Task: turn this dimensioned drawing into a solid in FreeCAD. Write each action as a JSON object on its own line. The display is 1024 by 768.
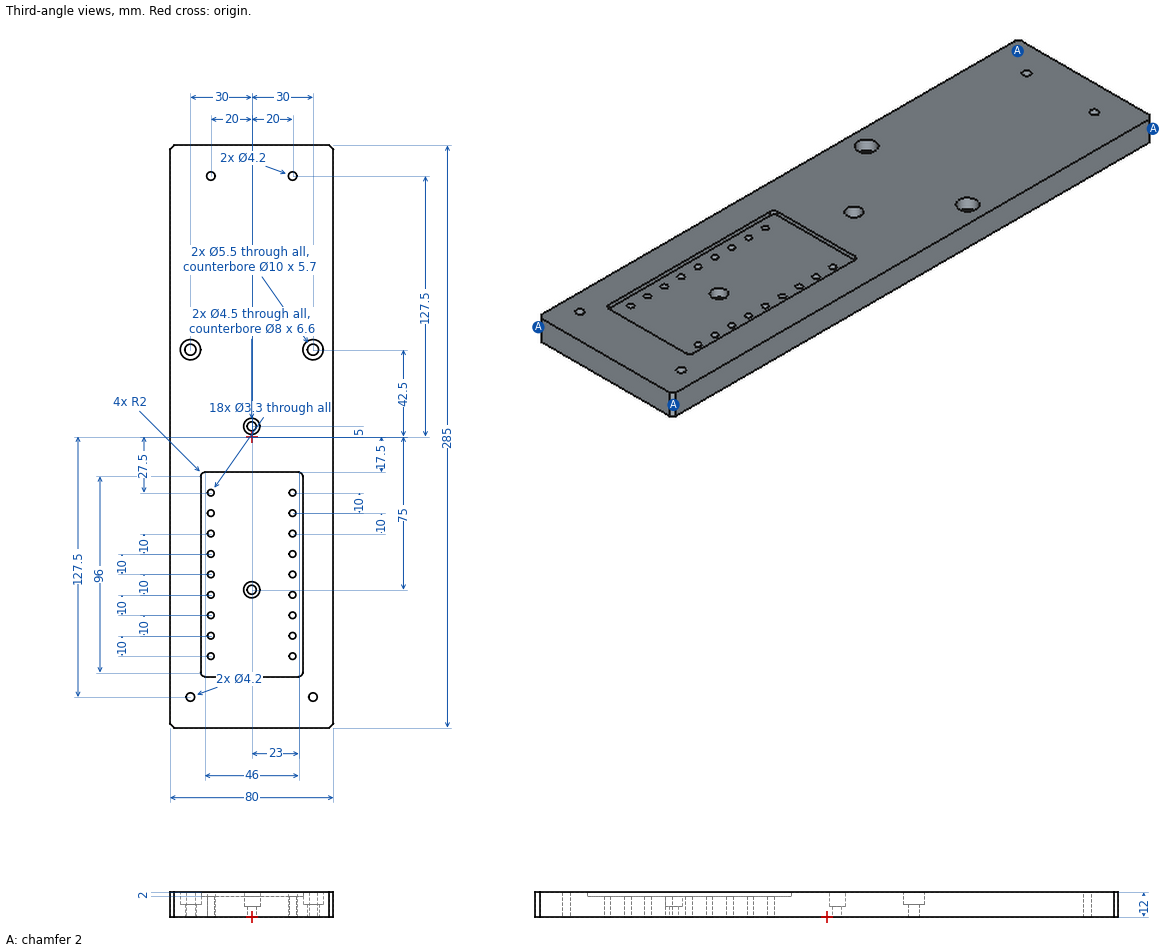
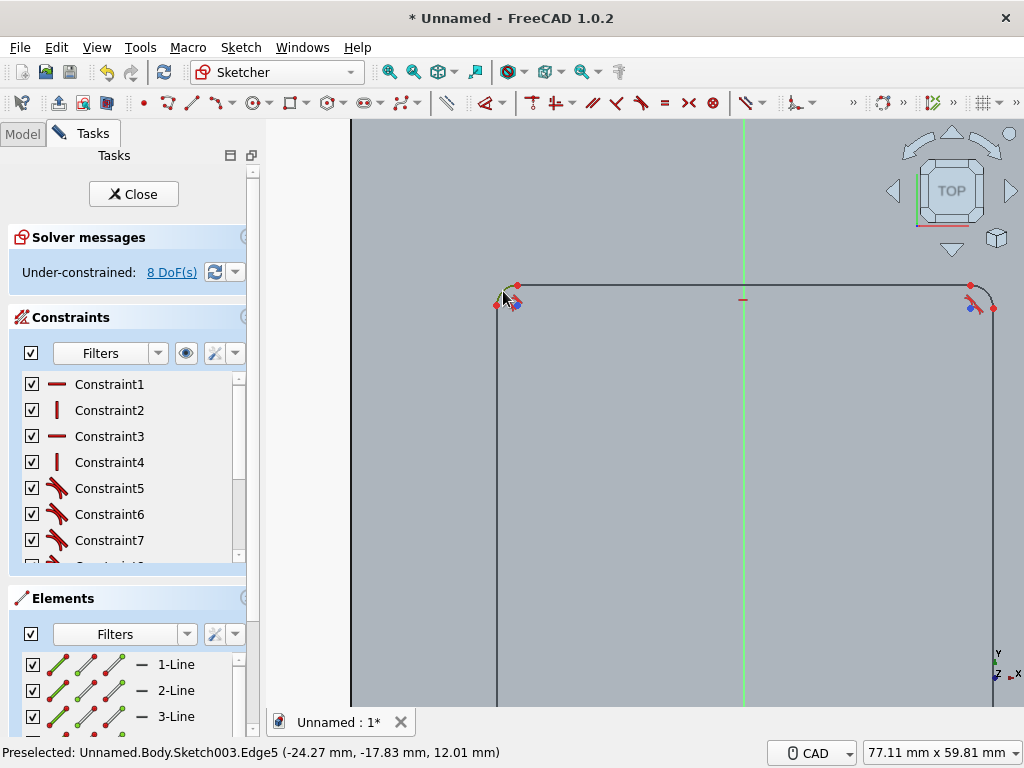
{"action": "scroll", "coordinate": [504, 293], "scroll_direction": "down", "scroll_amount": 6}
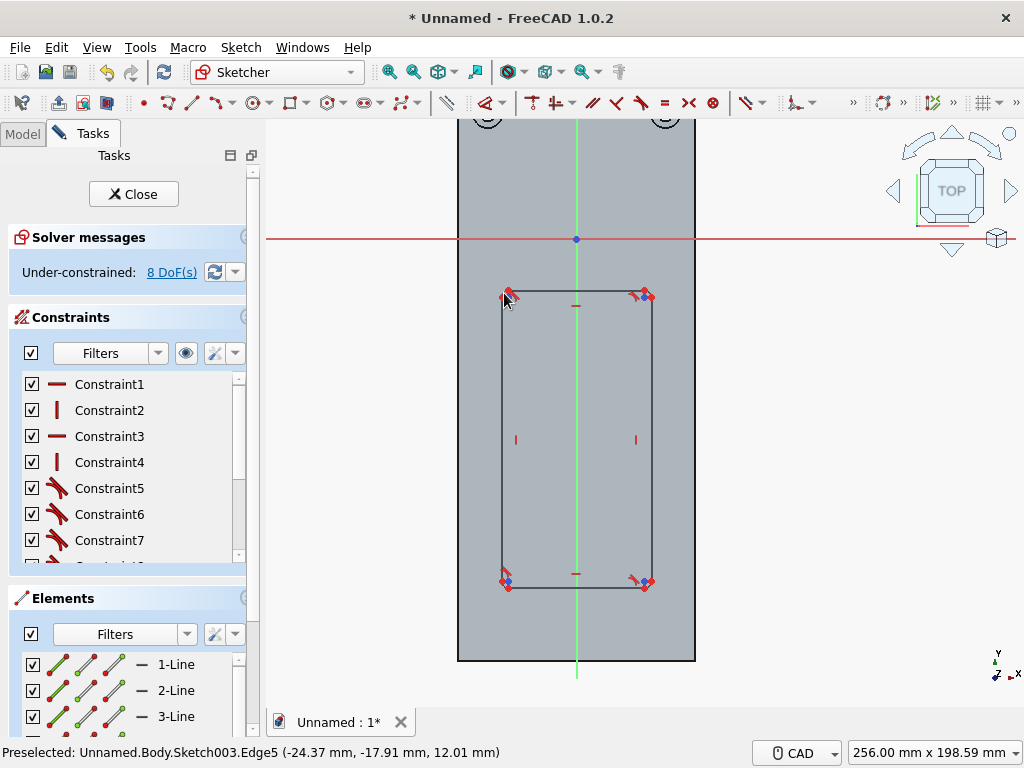
{"action": "scroll", "coordinate": [503, 585], "scroll_direction": "up", "scroll_amount": 8}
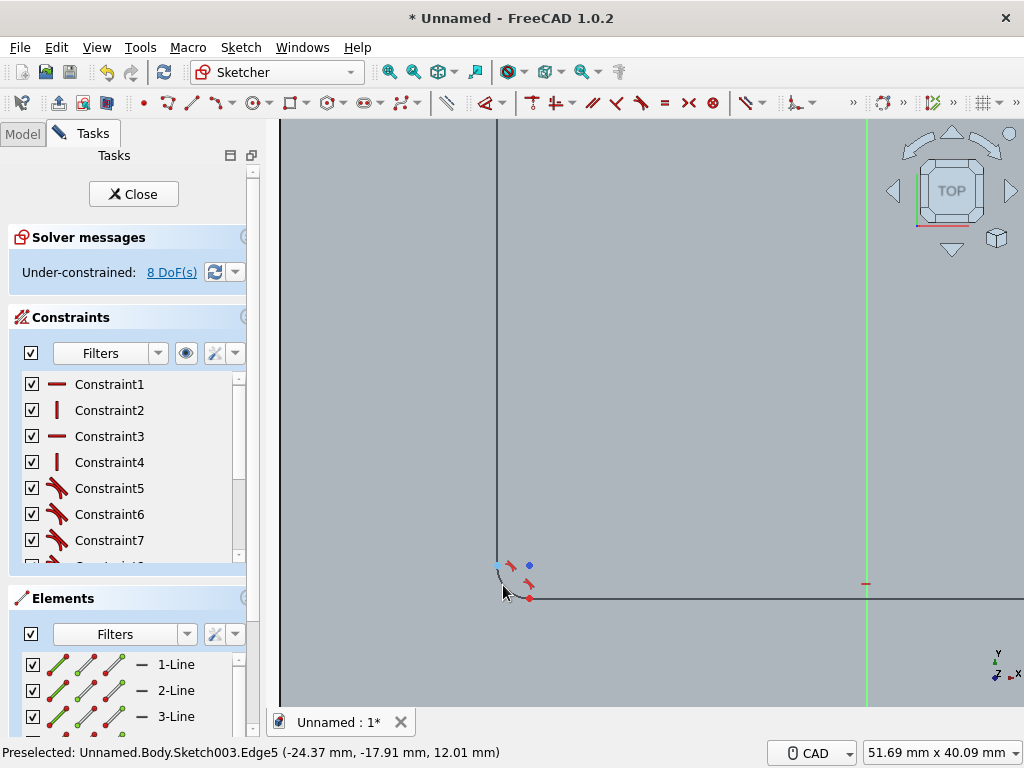
{"action": "left_click", "coordinate": [501, 581]}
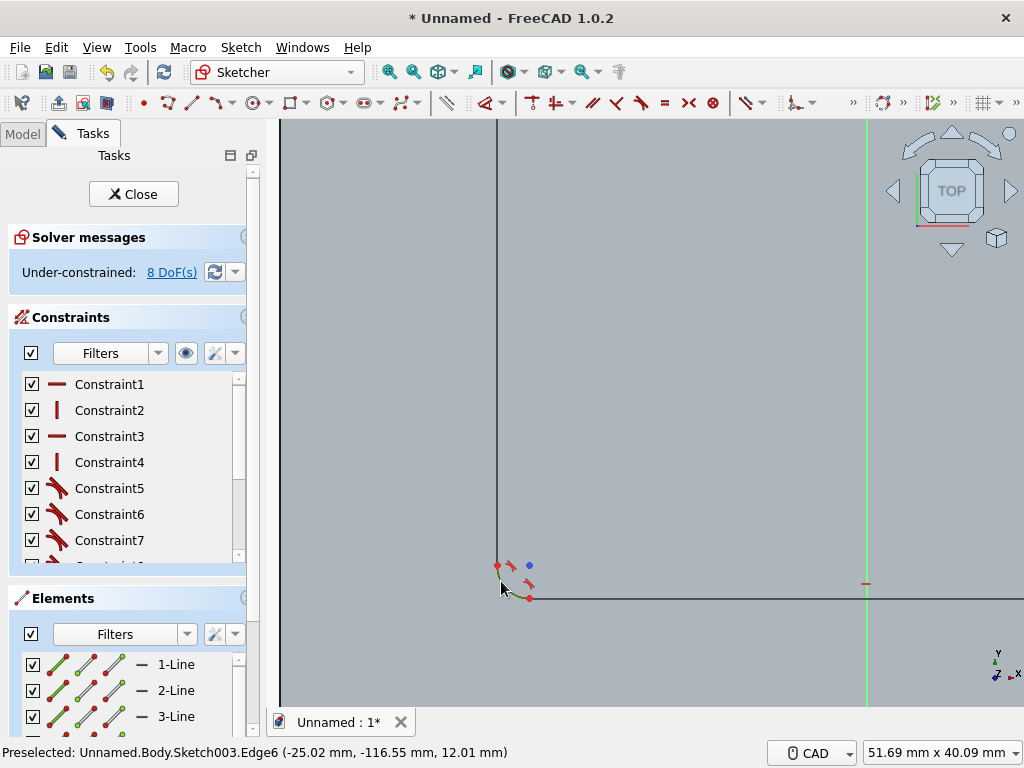
{"action": "scroll", "coordinate": [503, 586], "scroll_direction": "down", "scroll_amount": 8}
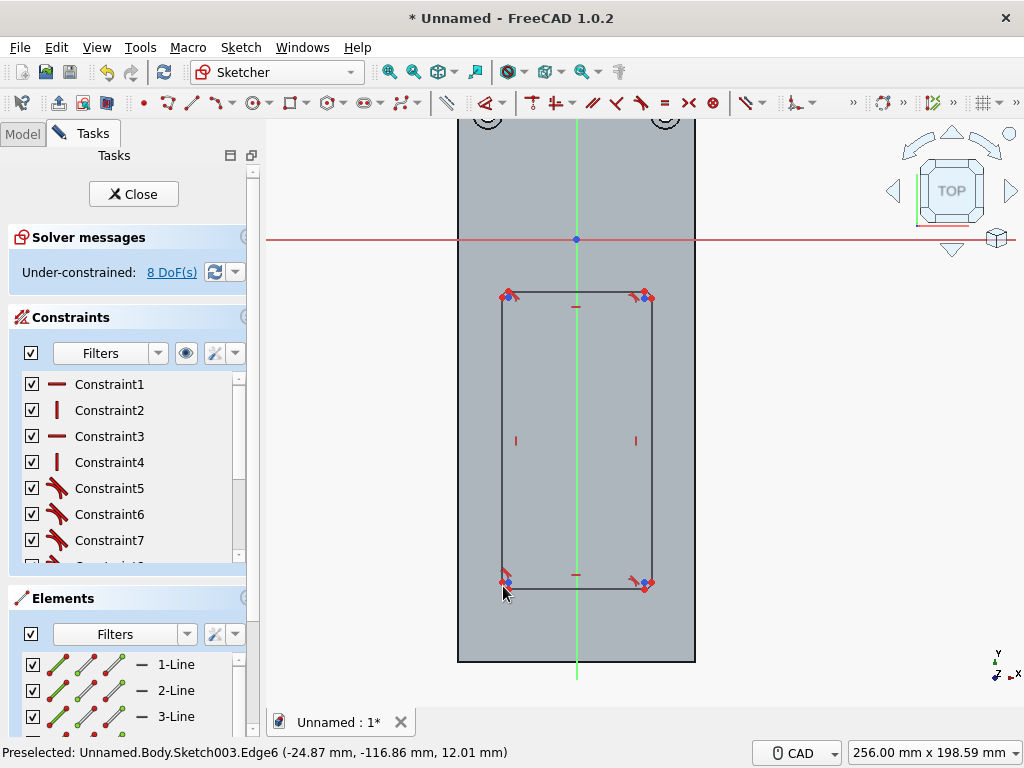
{"action": "scroll", "coordinate": [648, 588], "scroll_direction": "up", "scroll_amount": 8}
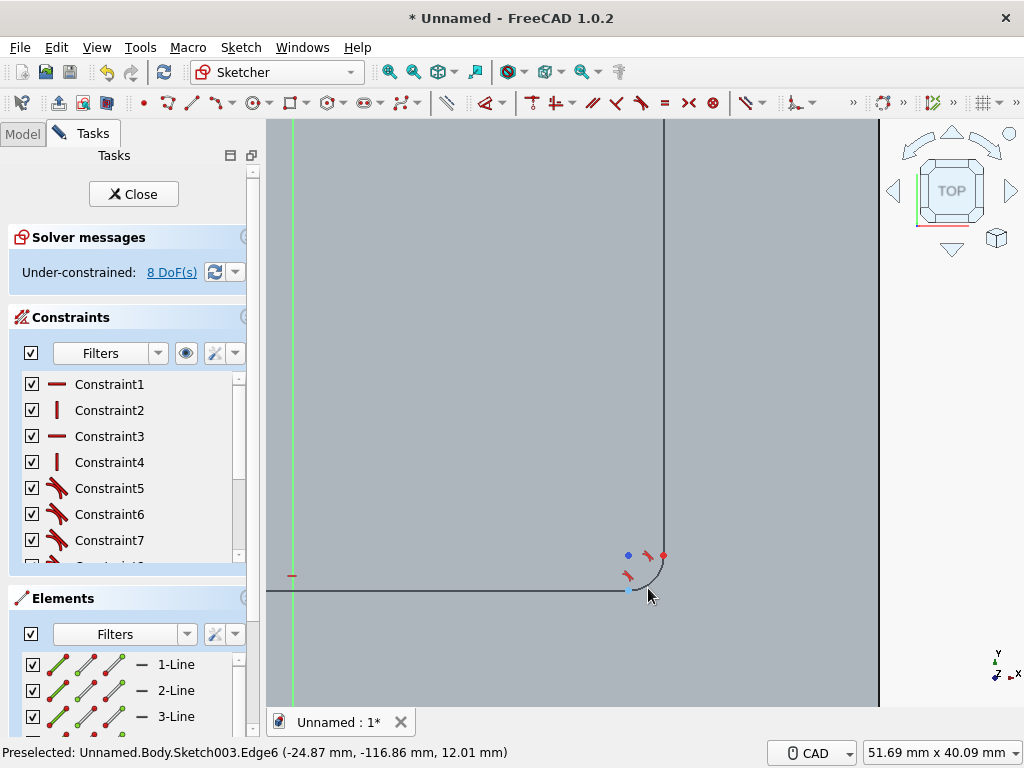
{"action": "left_click", "coordinate": [645, 587]}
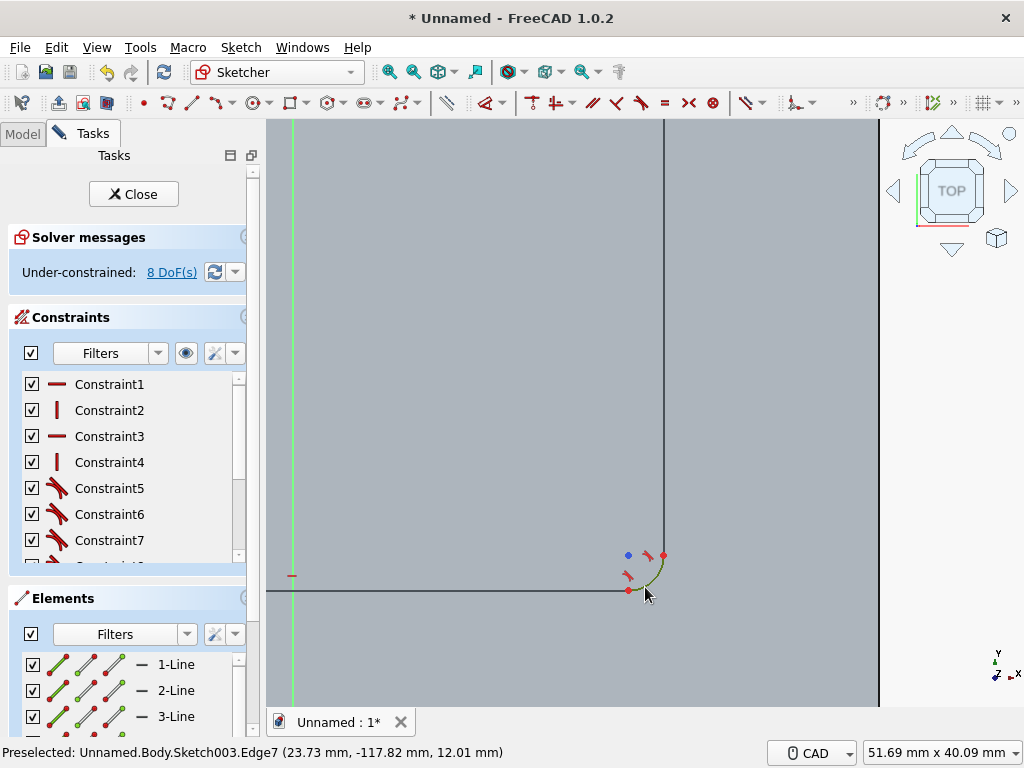
{"action": "scroll", "coordinate": [648, 588], "scroll_direction": "down", "scroll_amount": 8}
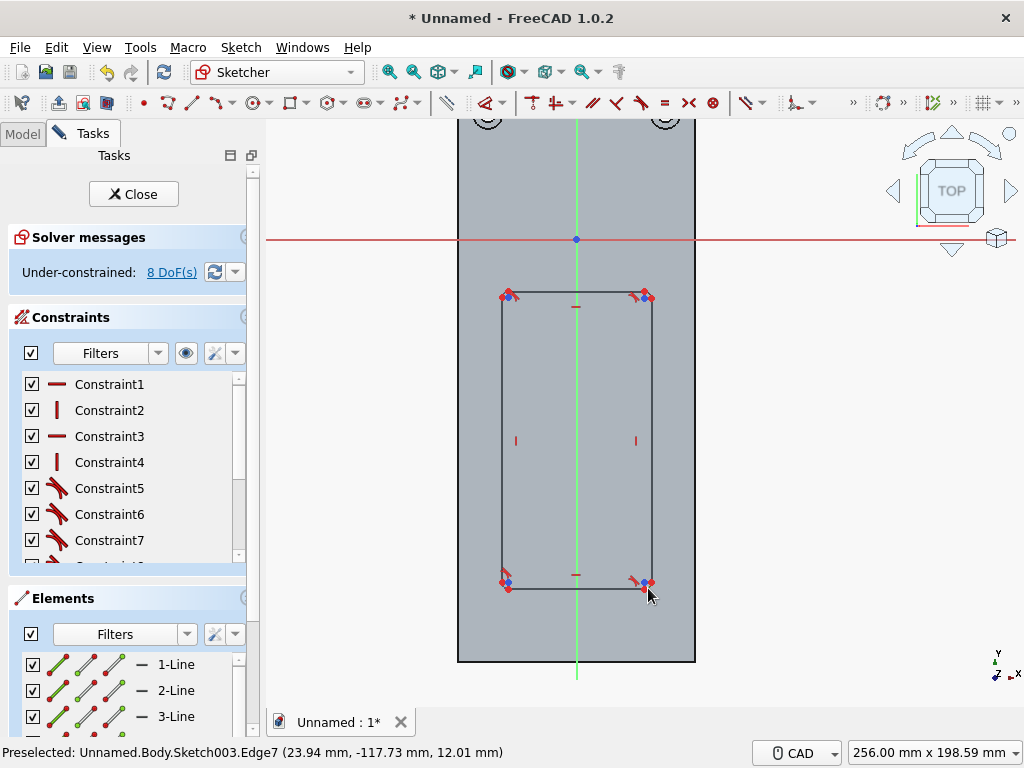
{"action": "scroll", "coordinate": [651, 295], "scroll_direction": "up", "scroll_amount": 8}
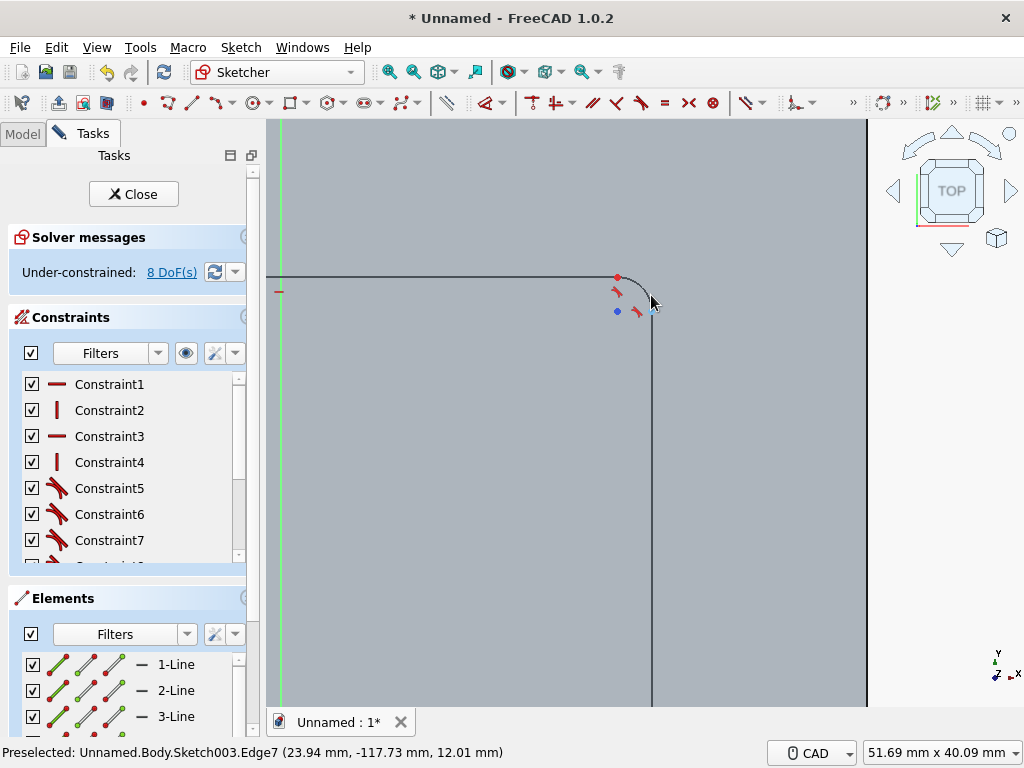
{"action": "left_click", "coordinate": [648, 296]}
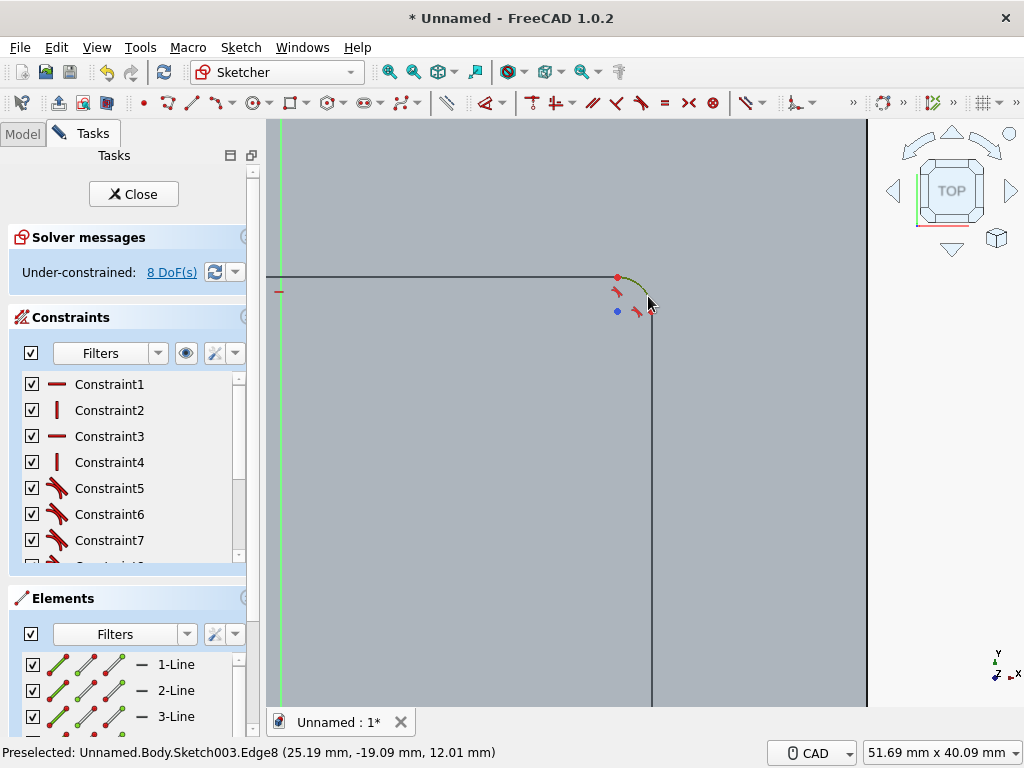
{"action": "key", "text": "e"}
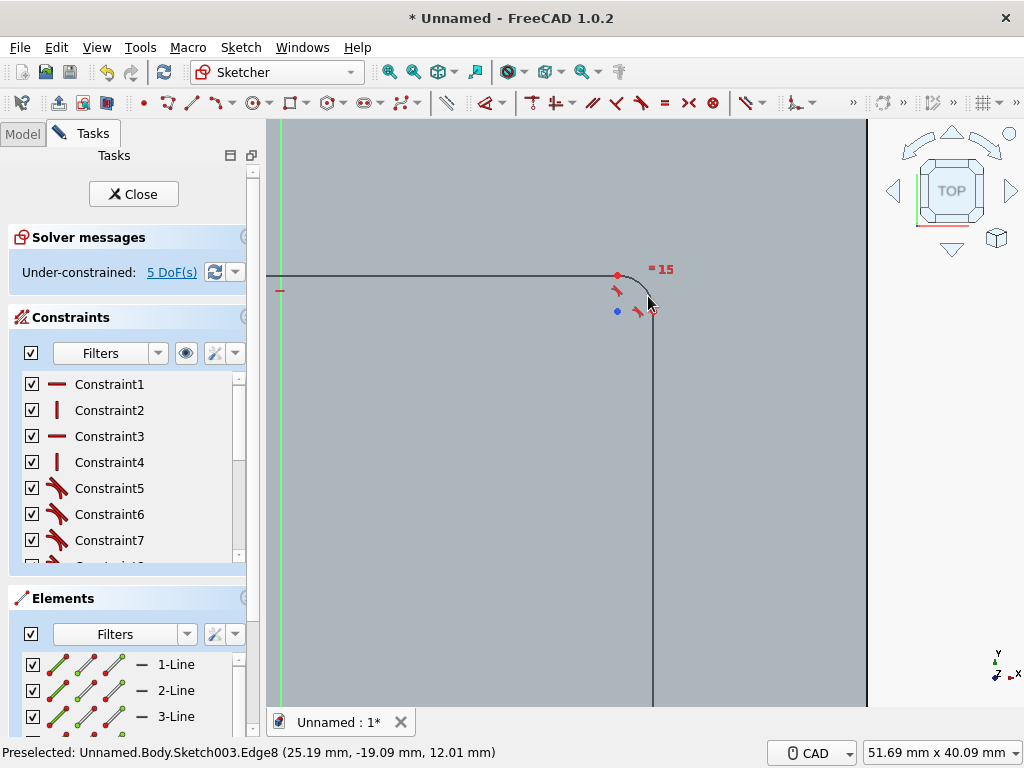
{"action": "key", "text": "d"}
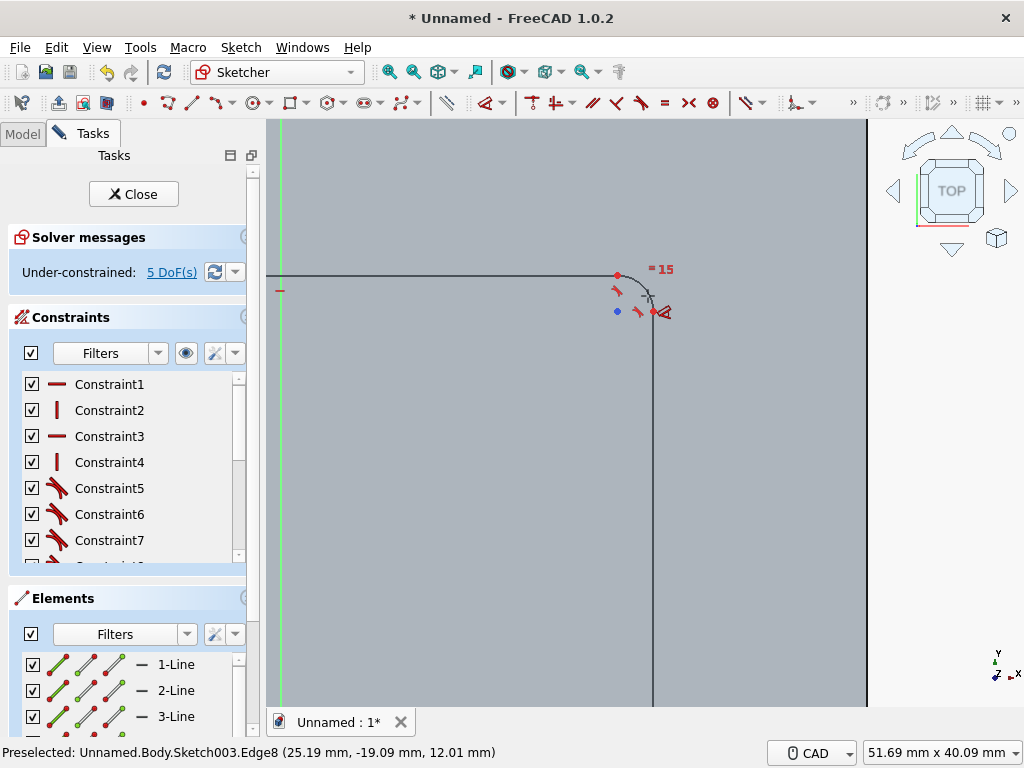
{"action": "scroll", "coordinate": [651, 294], "scroll_direction": "down", "scroll_amount": 8}